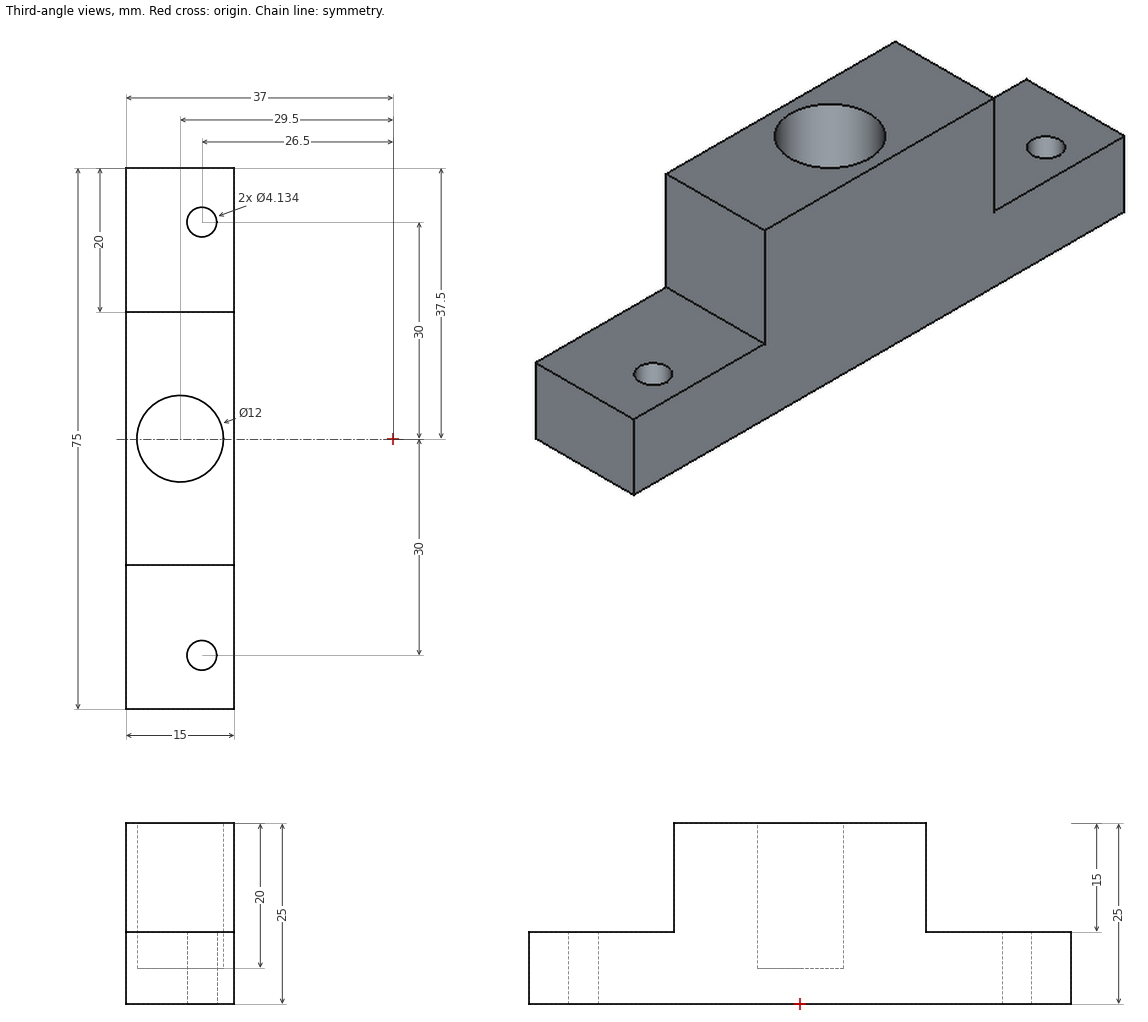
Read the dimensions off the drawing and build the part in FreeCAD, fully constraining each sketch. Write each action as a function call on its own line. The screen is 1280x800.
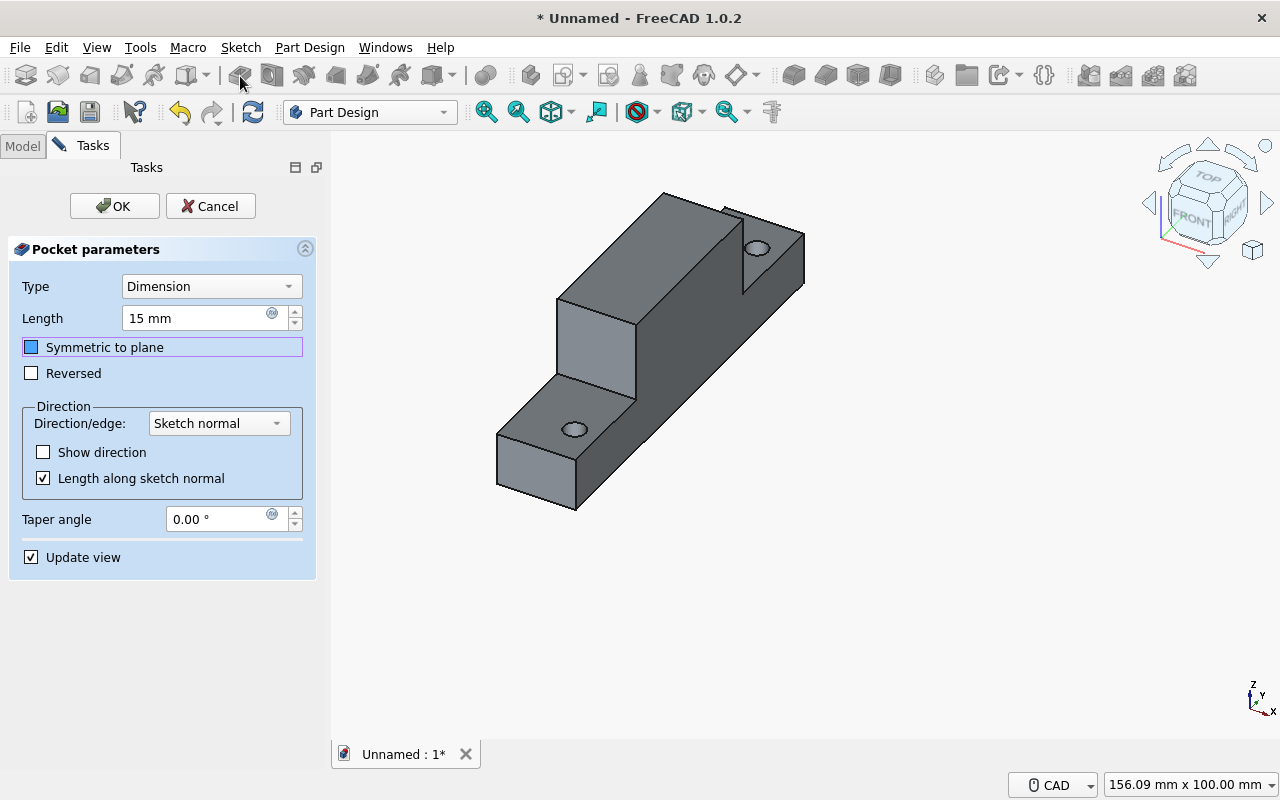
click(115, 206)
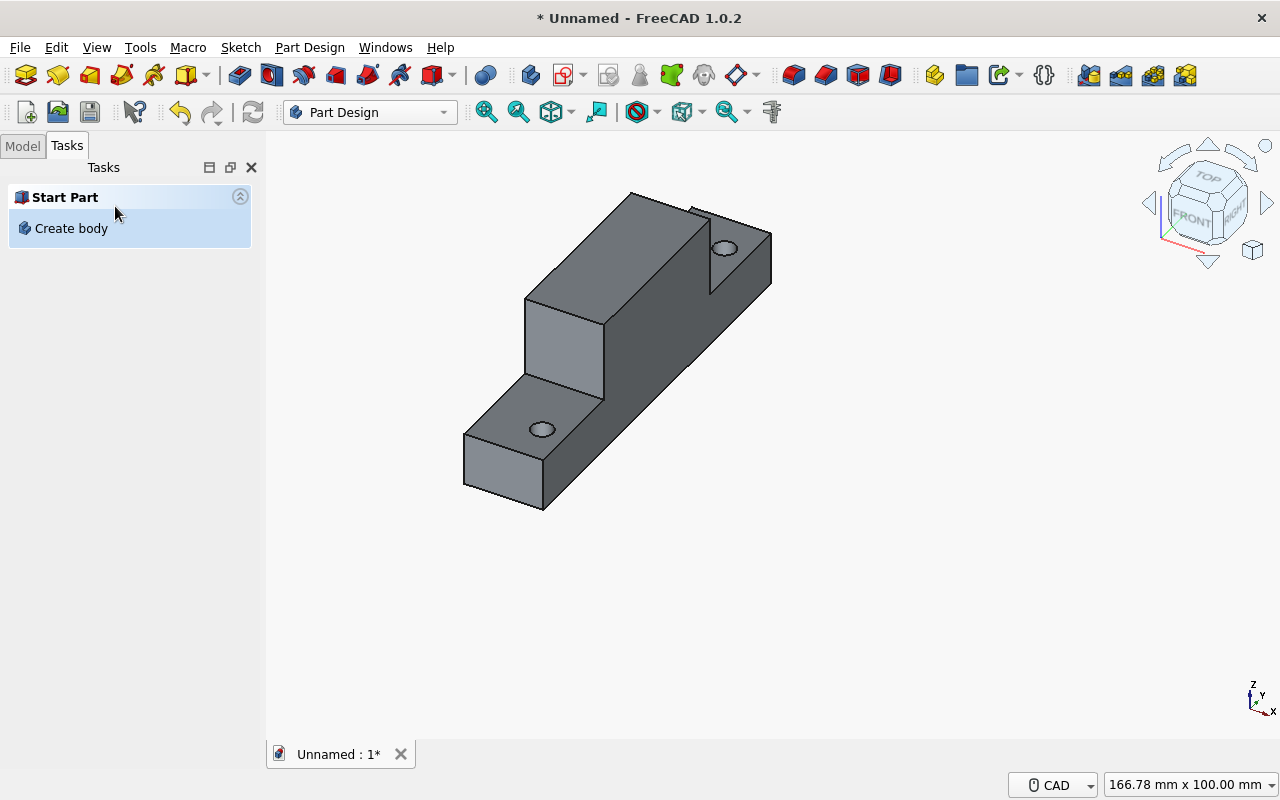
click(648, 228)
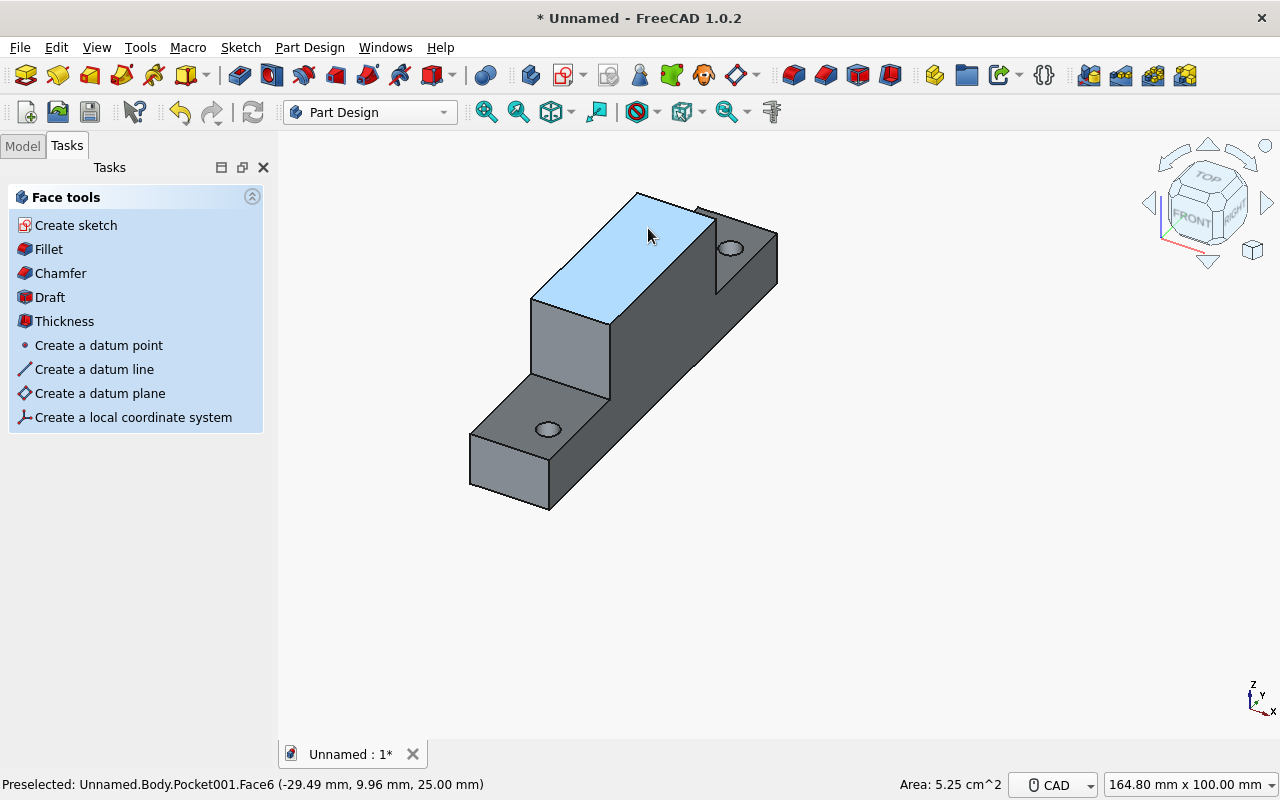
click(564, 76)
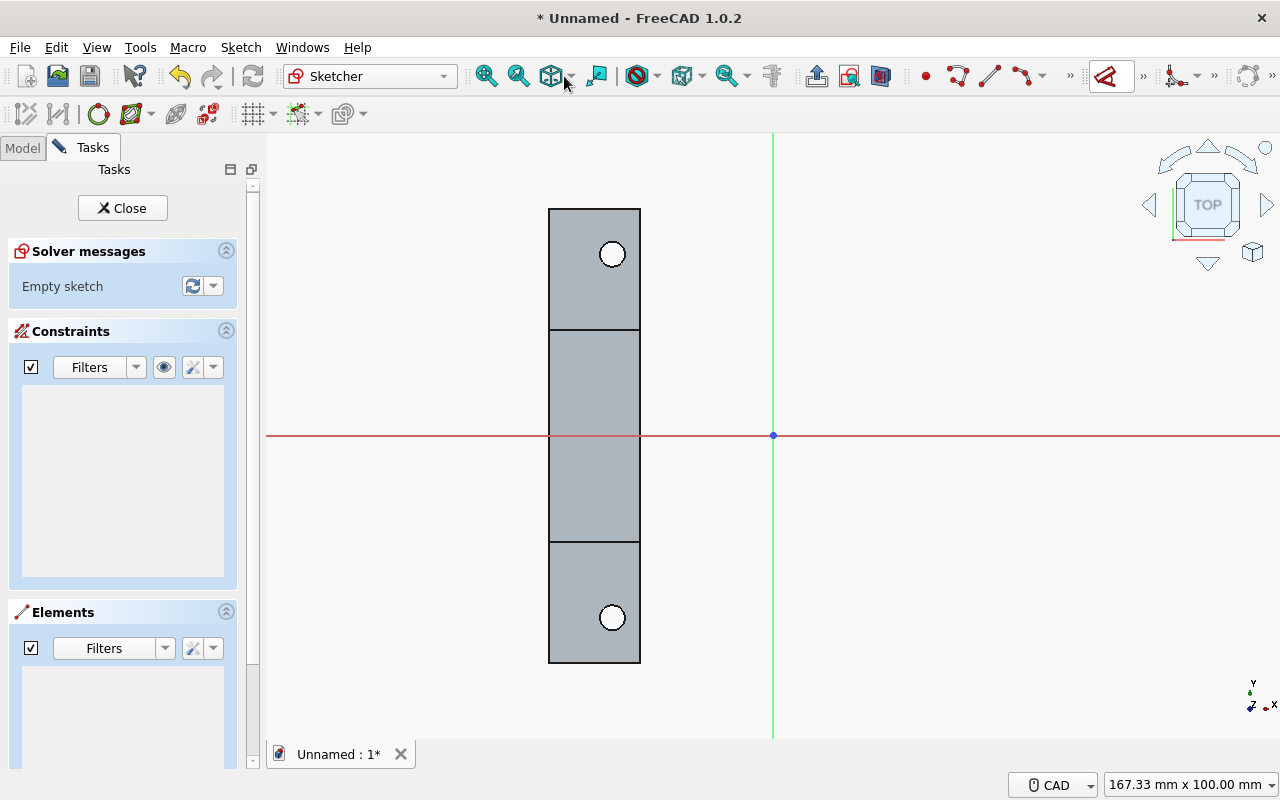
scroll(566, 436, up, 8)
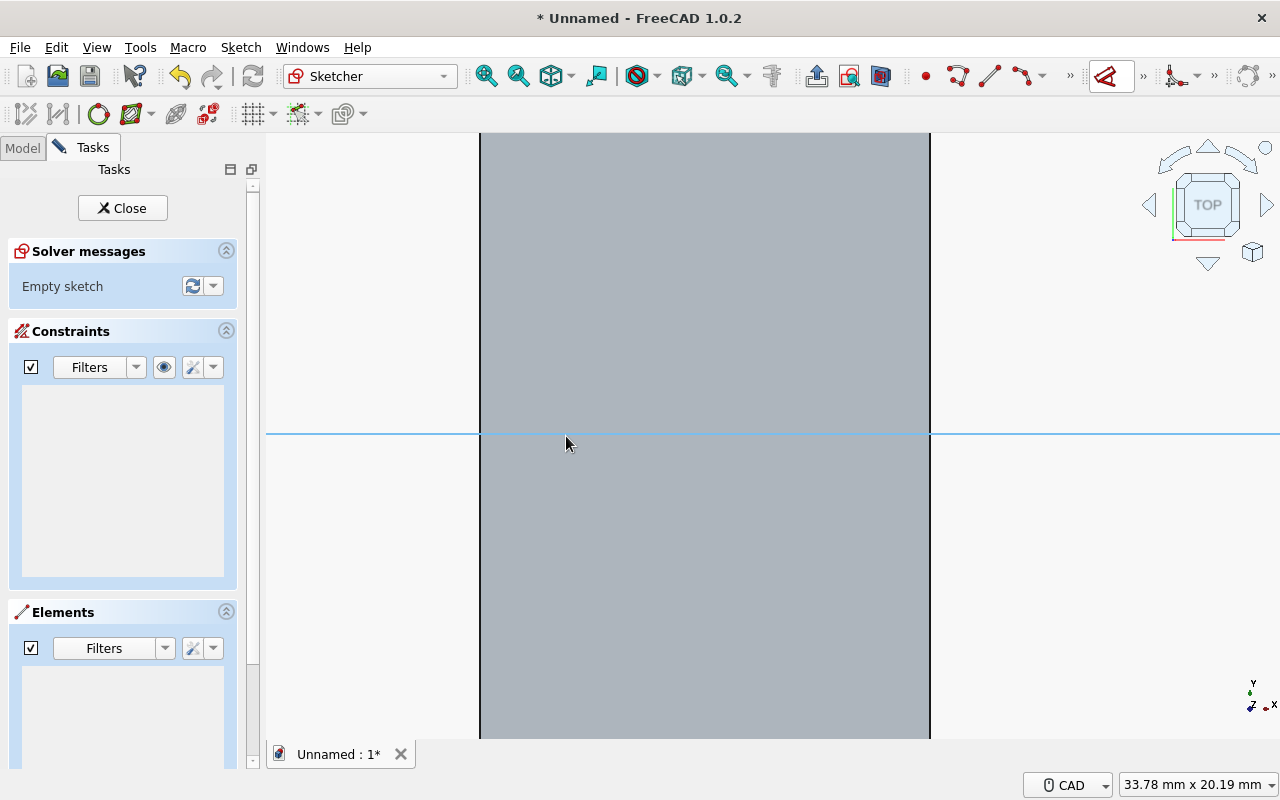
key(g)
key(c)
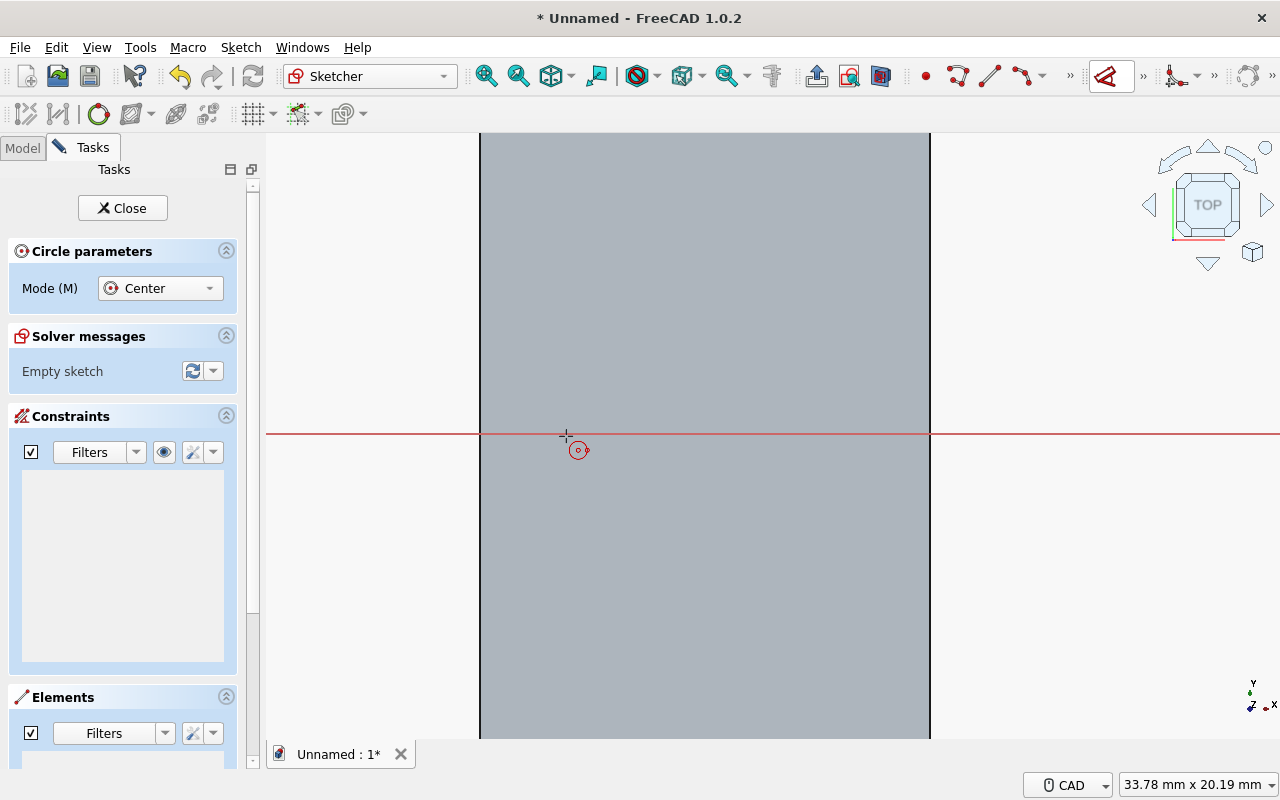
click(705, 434)
click(832, 307)
key(Escape)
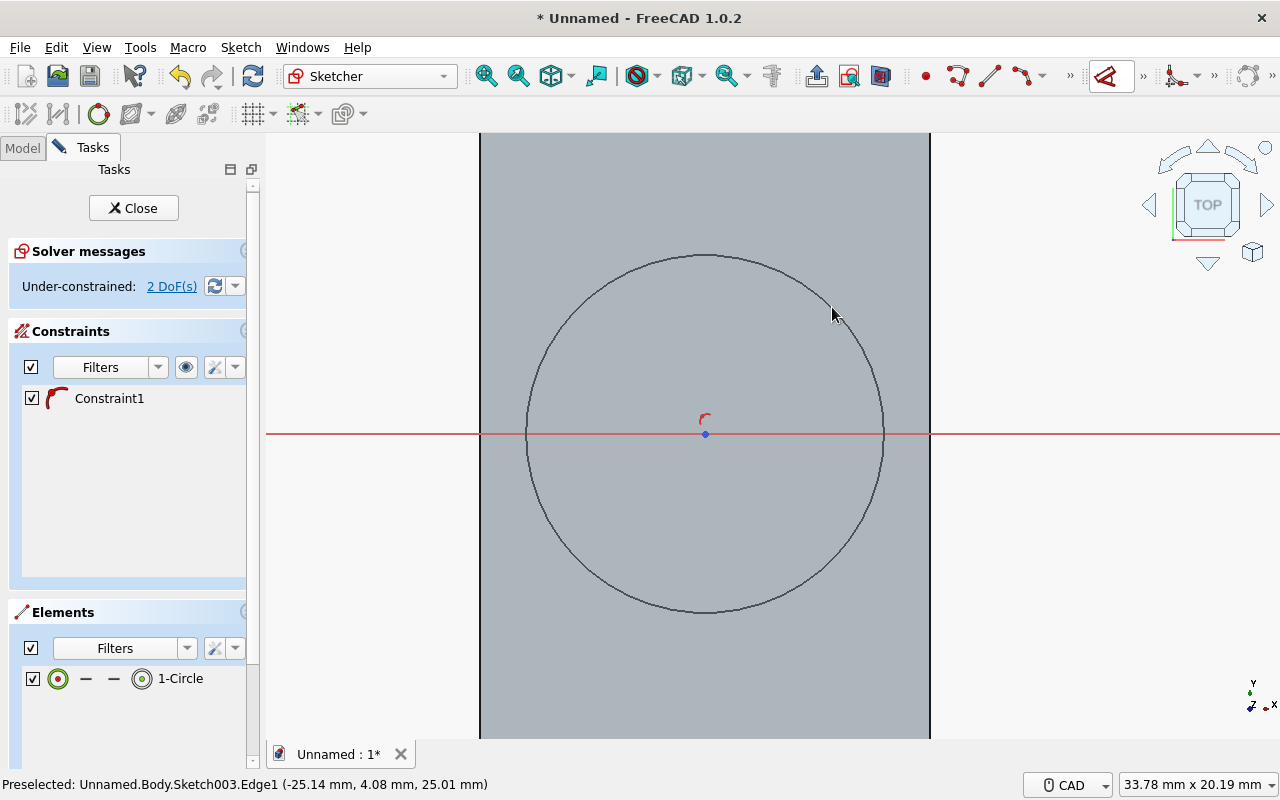
click(831, 307)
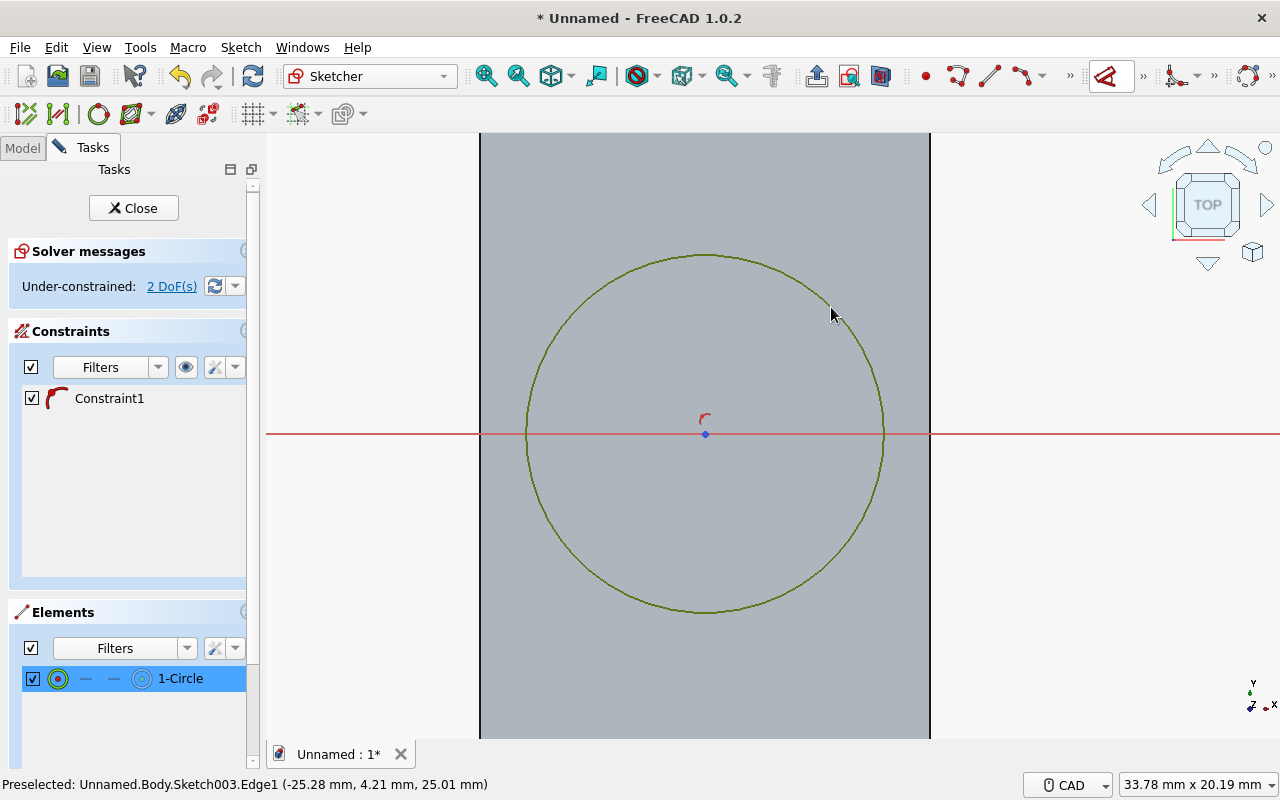
click(1128, 76)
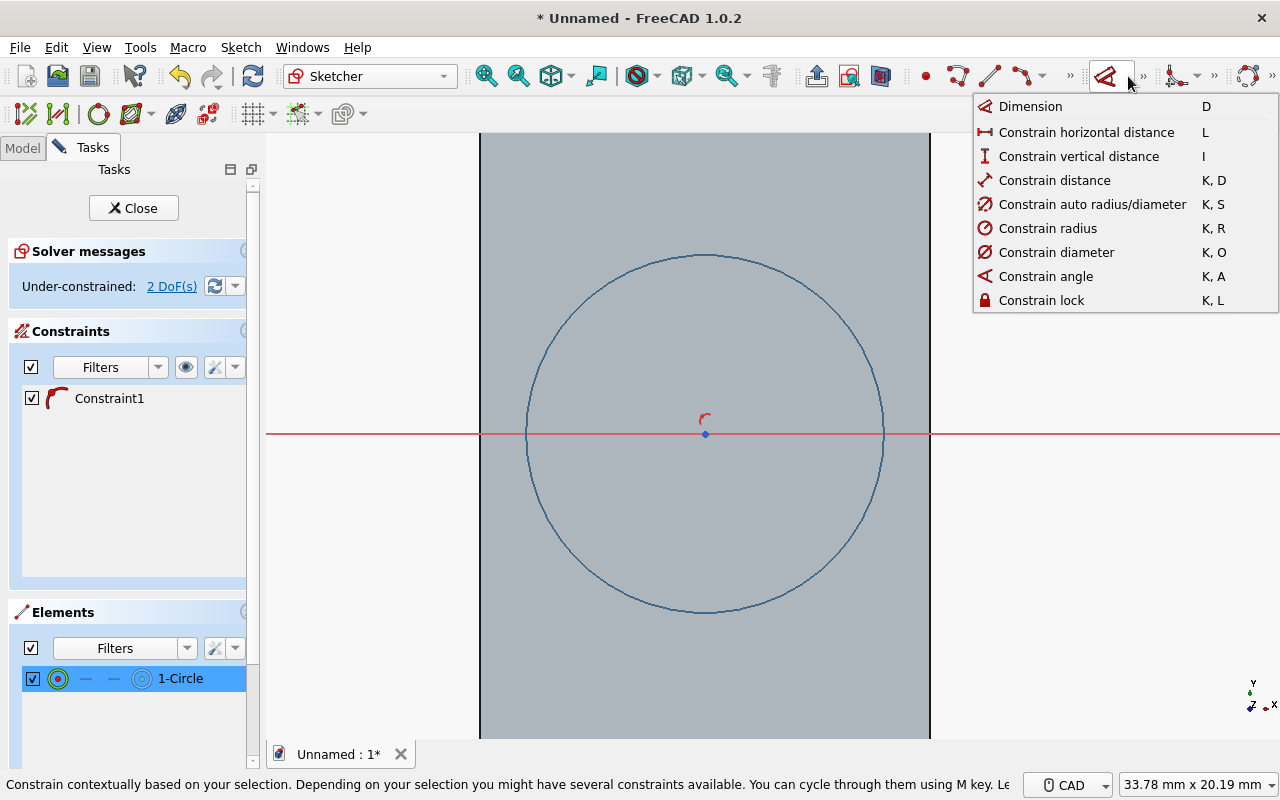
click(1126, 252)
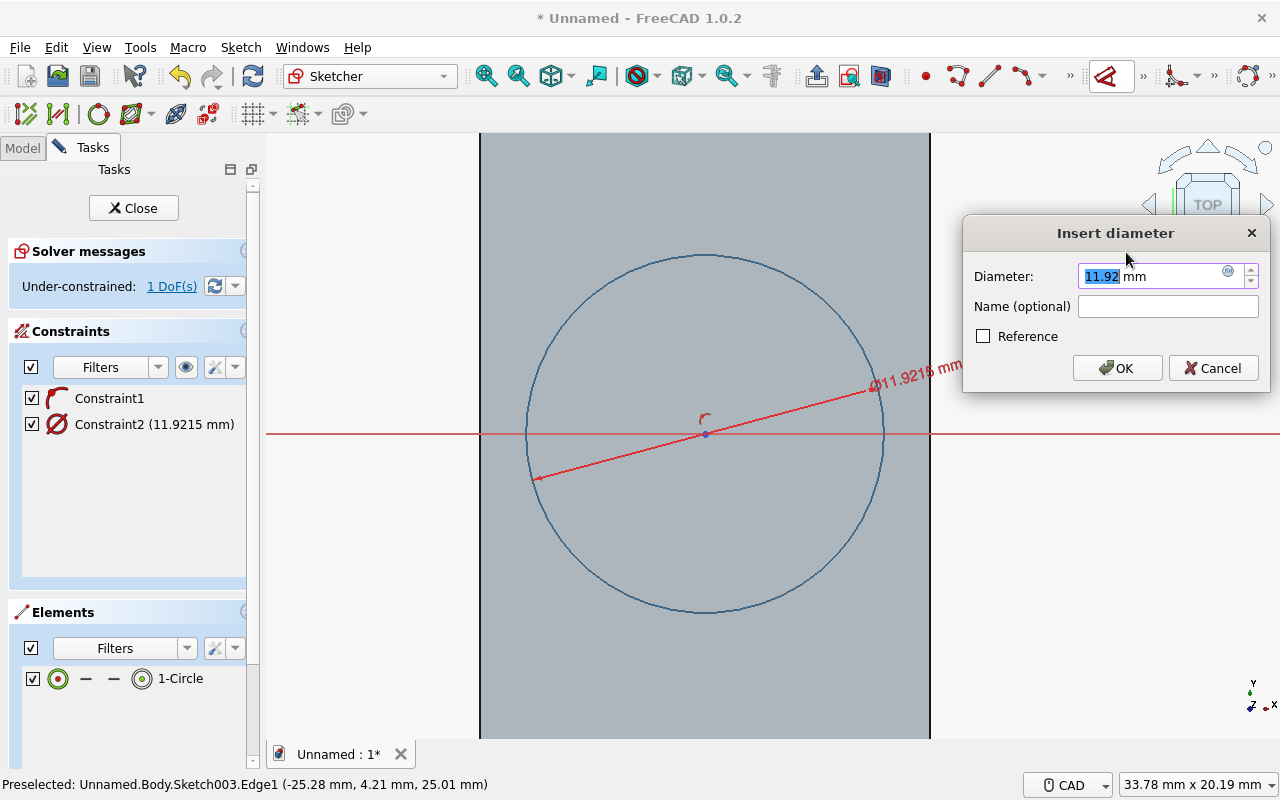
text(12)
key(Return)